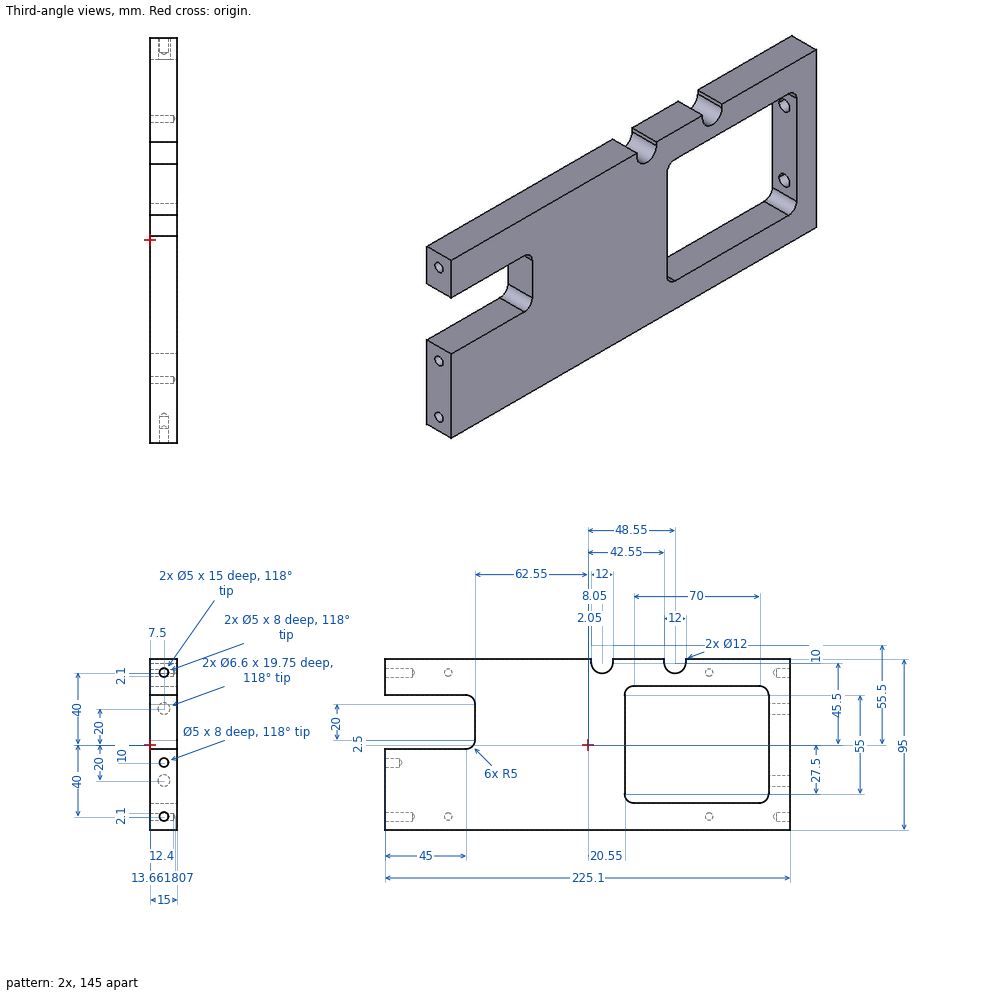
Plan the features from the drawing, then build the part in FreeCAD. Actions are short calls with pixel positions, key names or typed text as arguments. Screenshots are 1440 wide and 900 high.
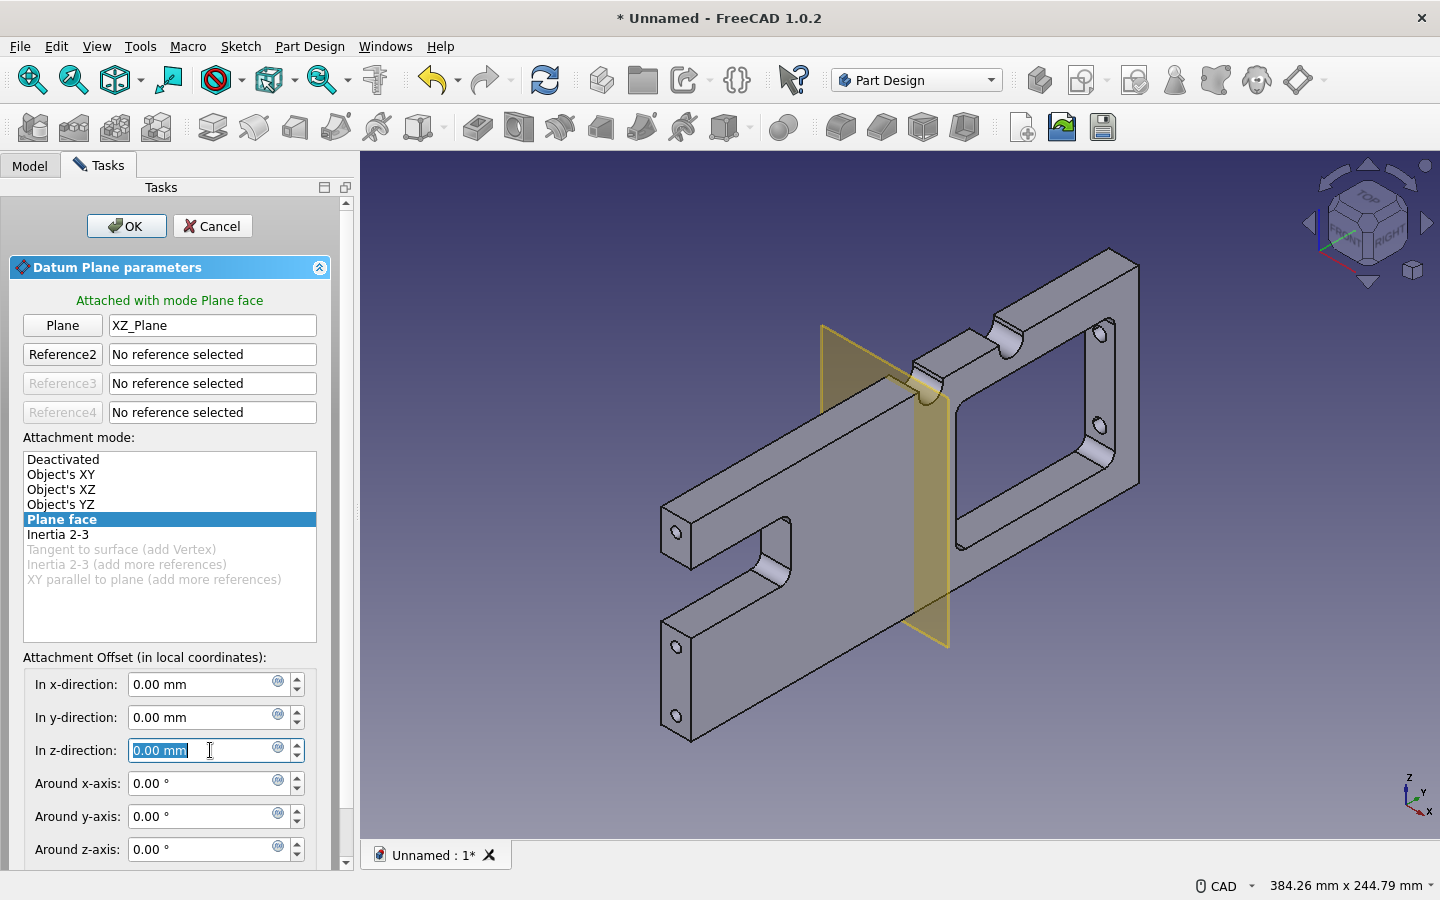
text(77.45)
key(Tab)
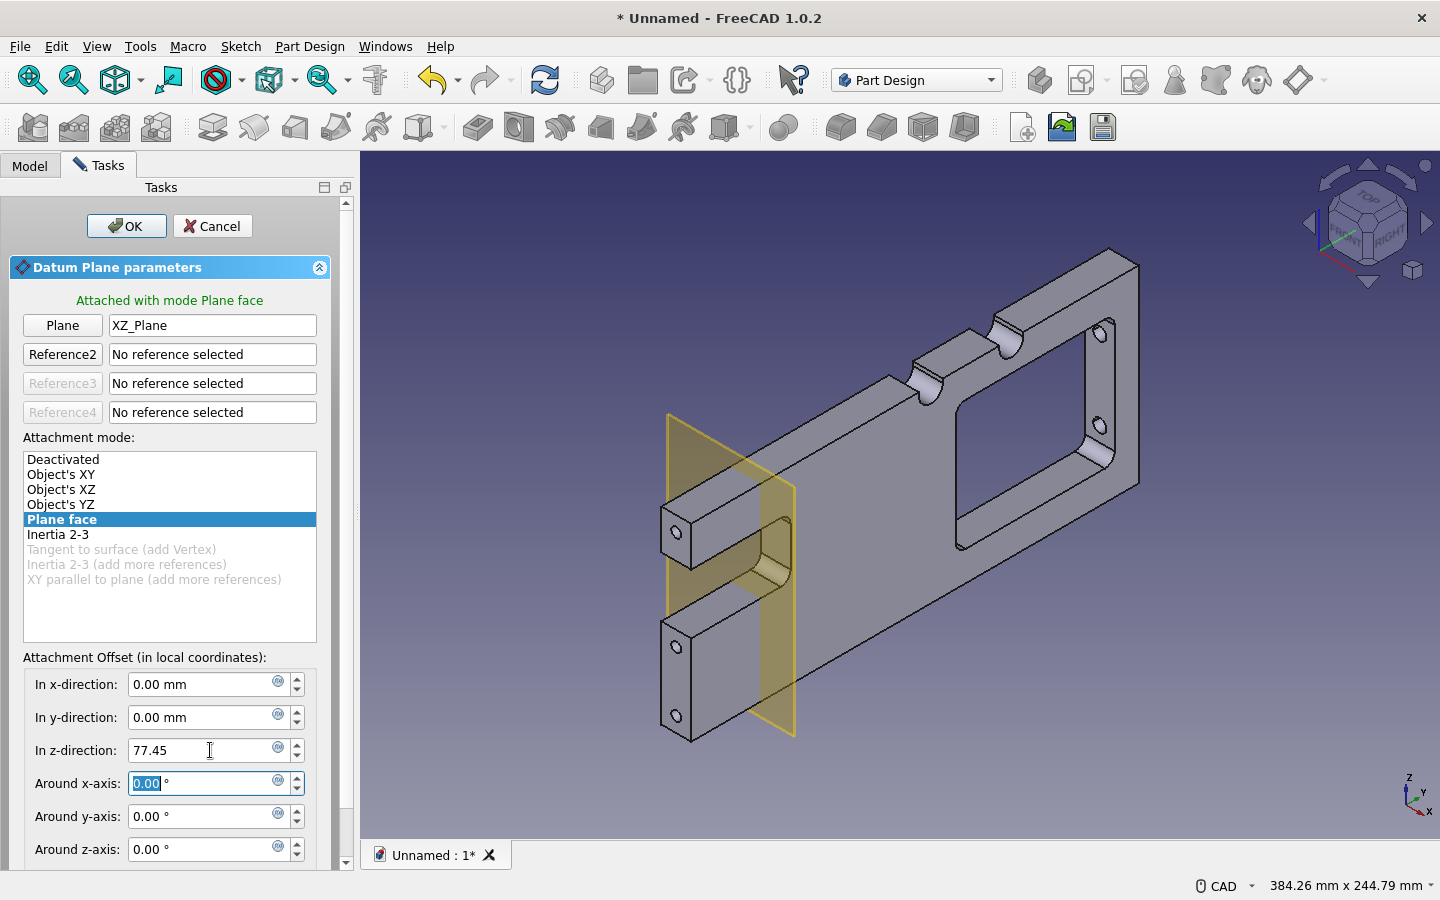
click(127, 226)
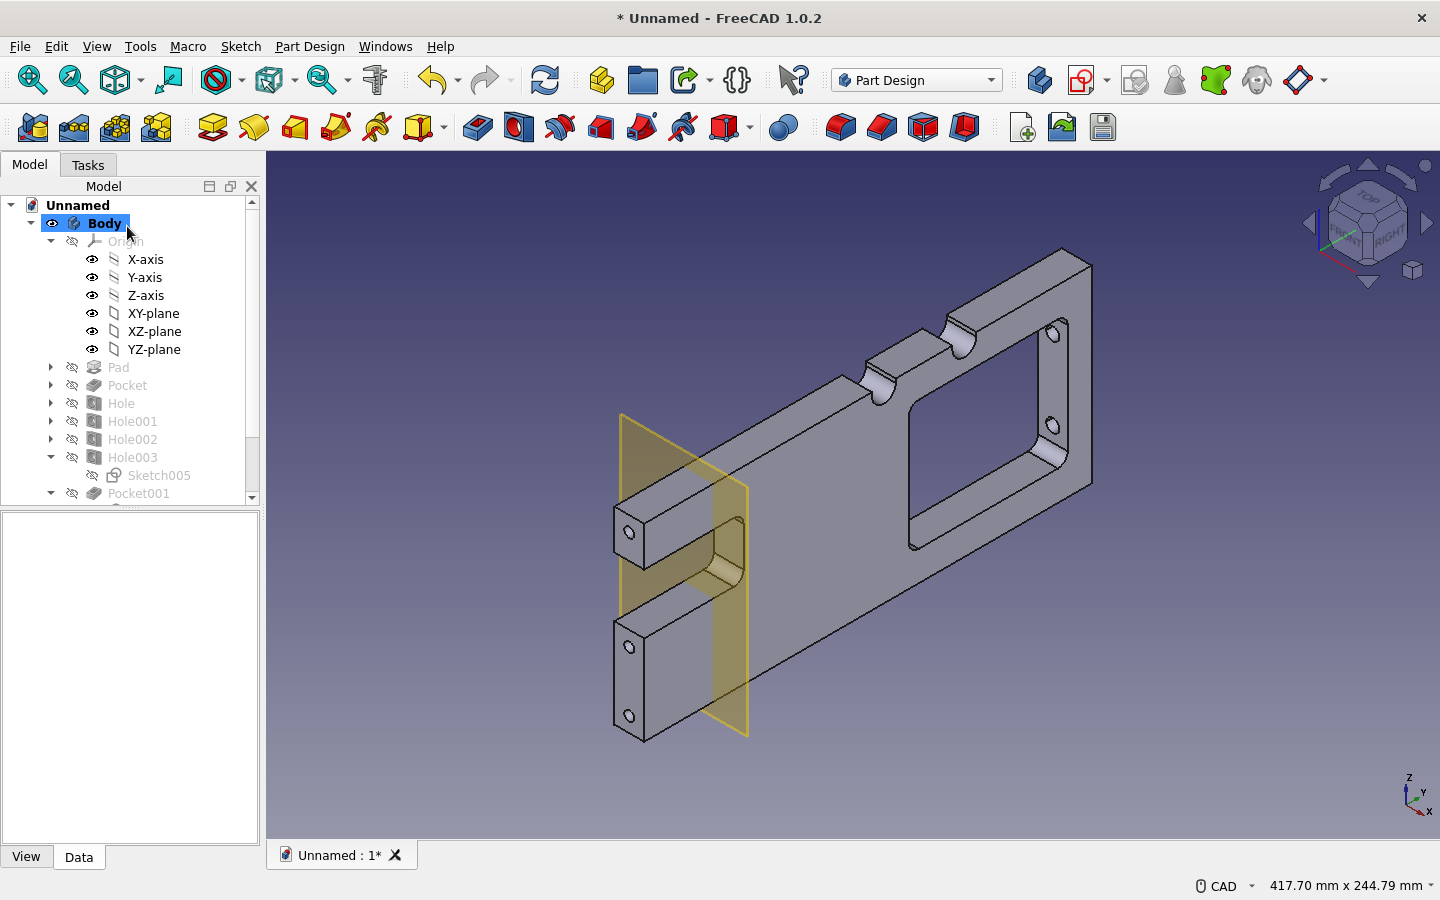
scroll(101, 345, down, 3)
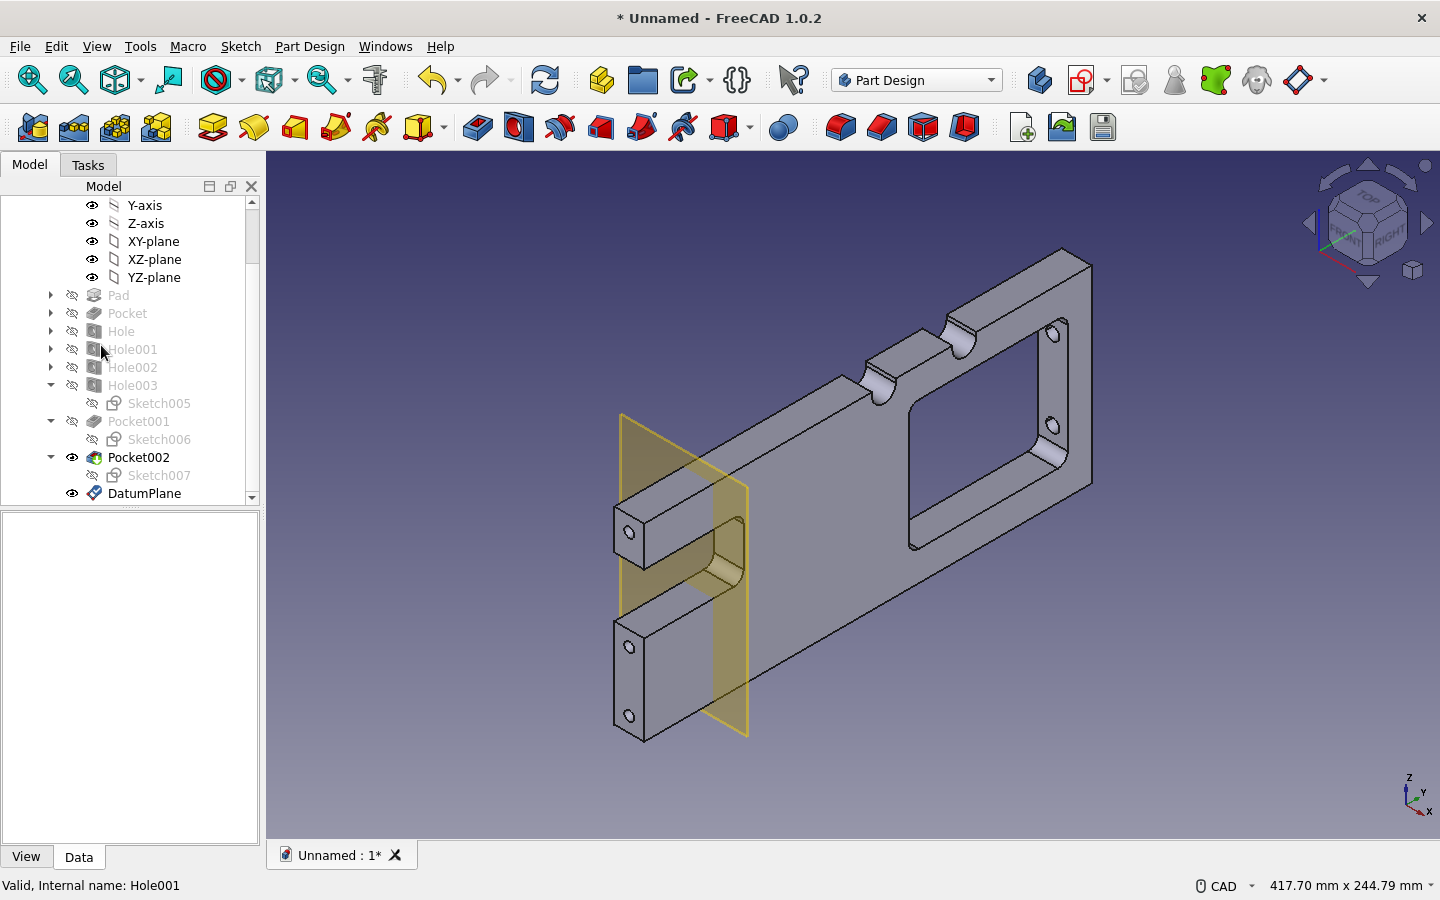
click(117, 493)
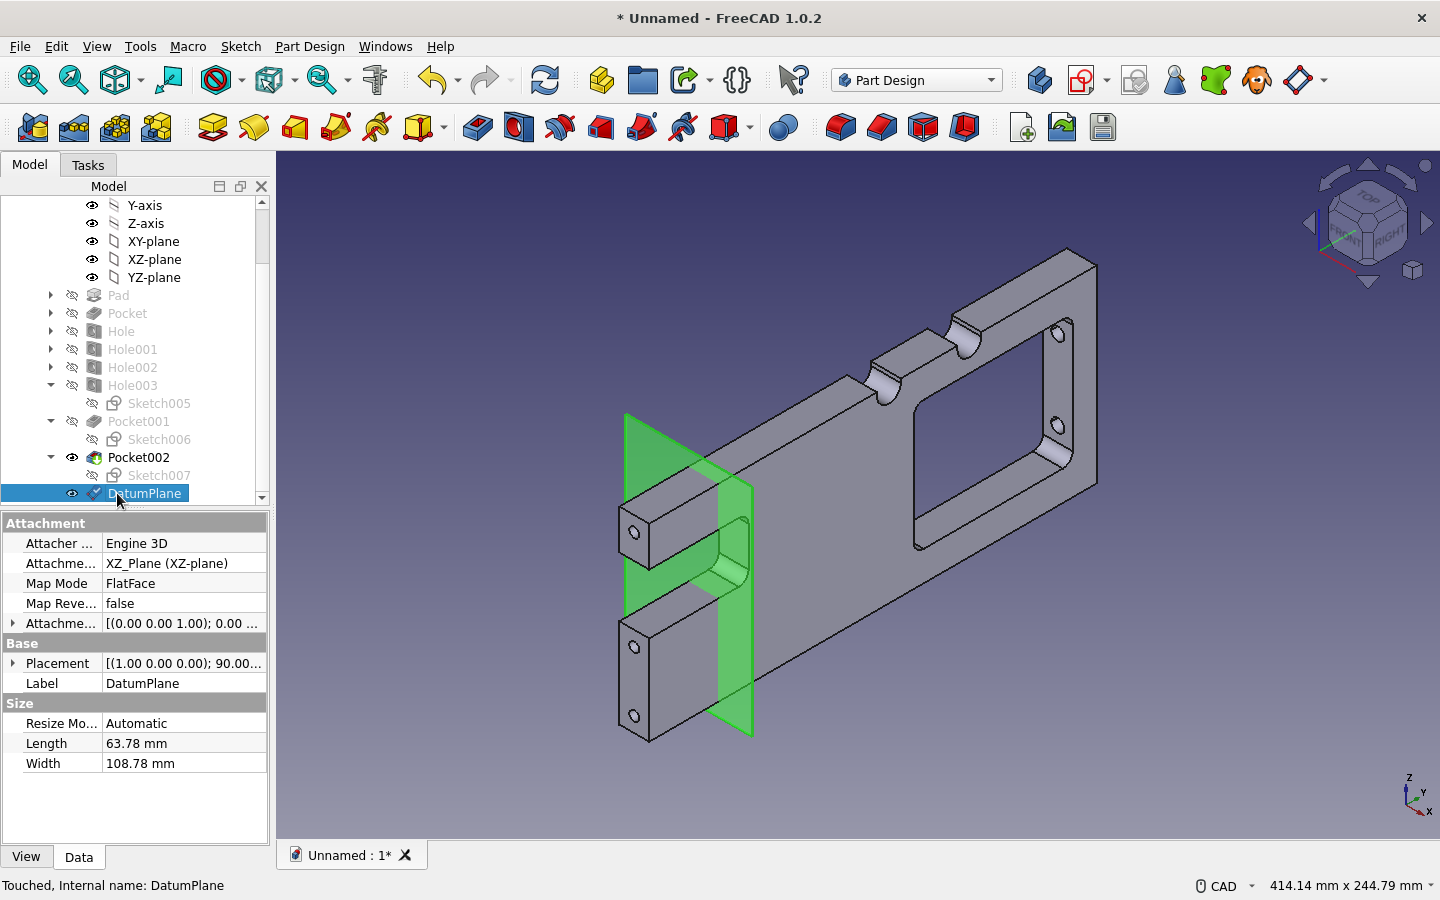
click(1080, 80)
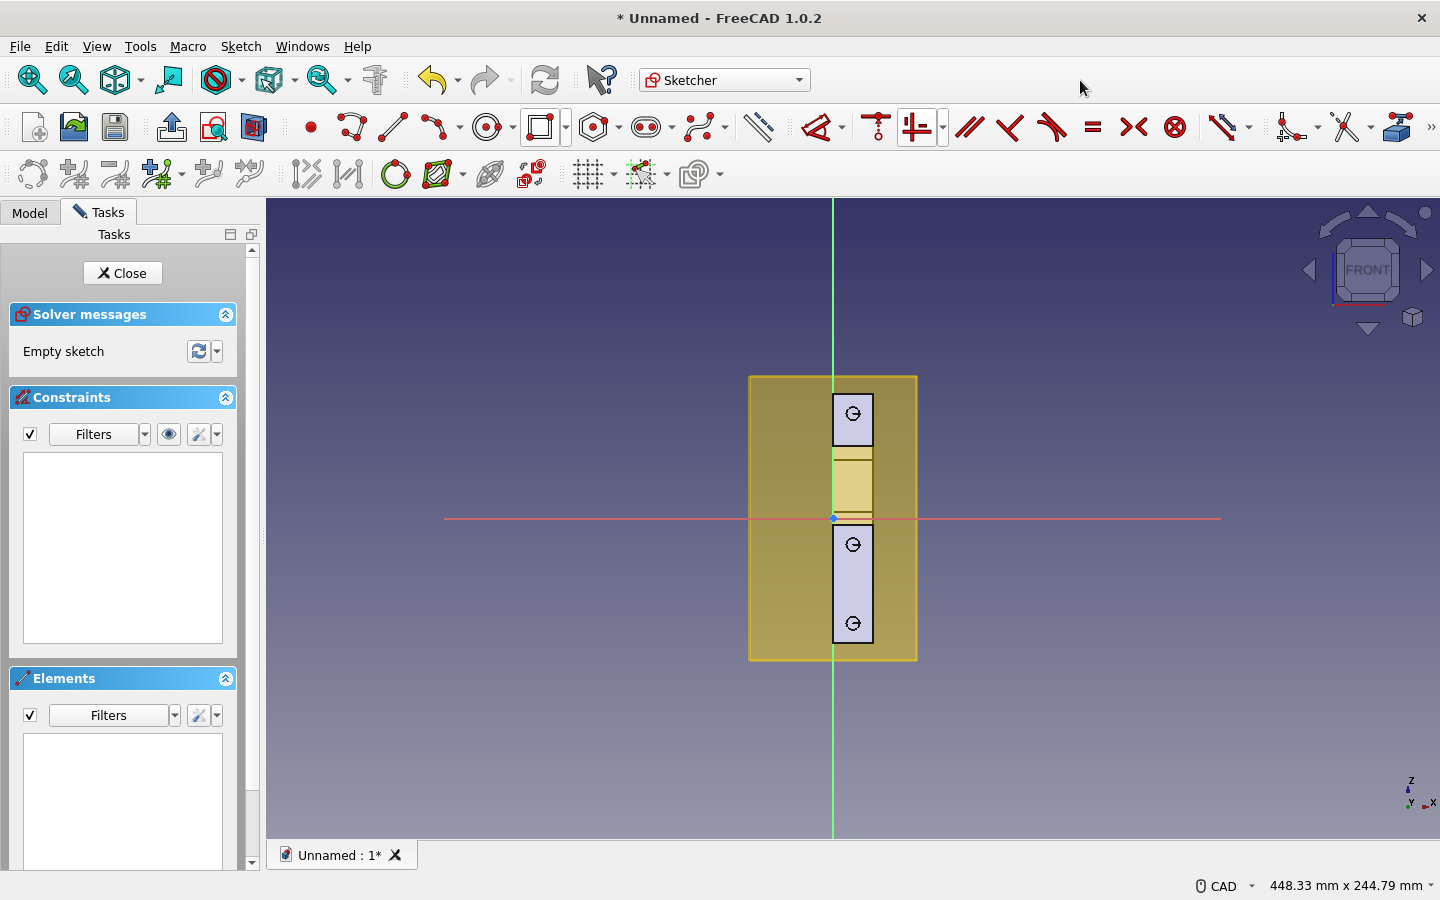
click(254, 128)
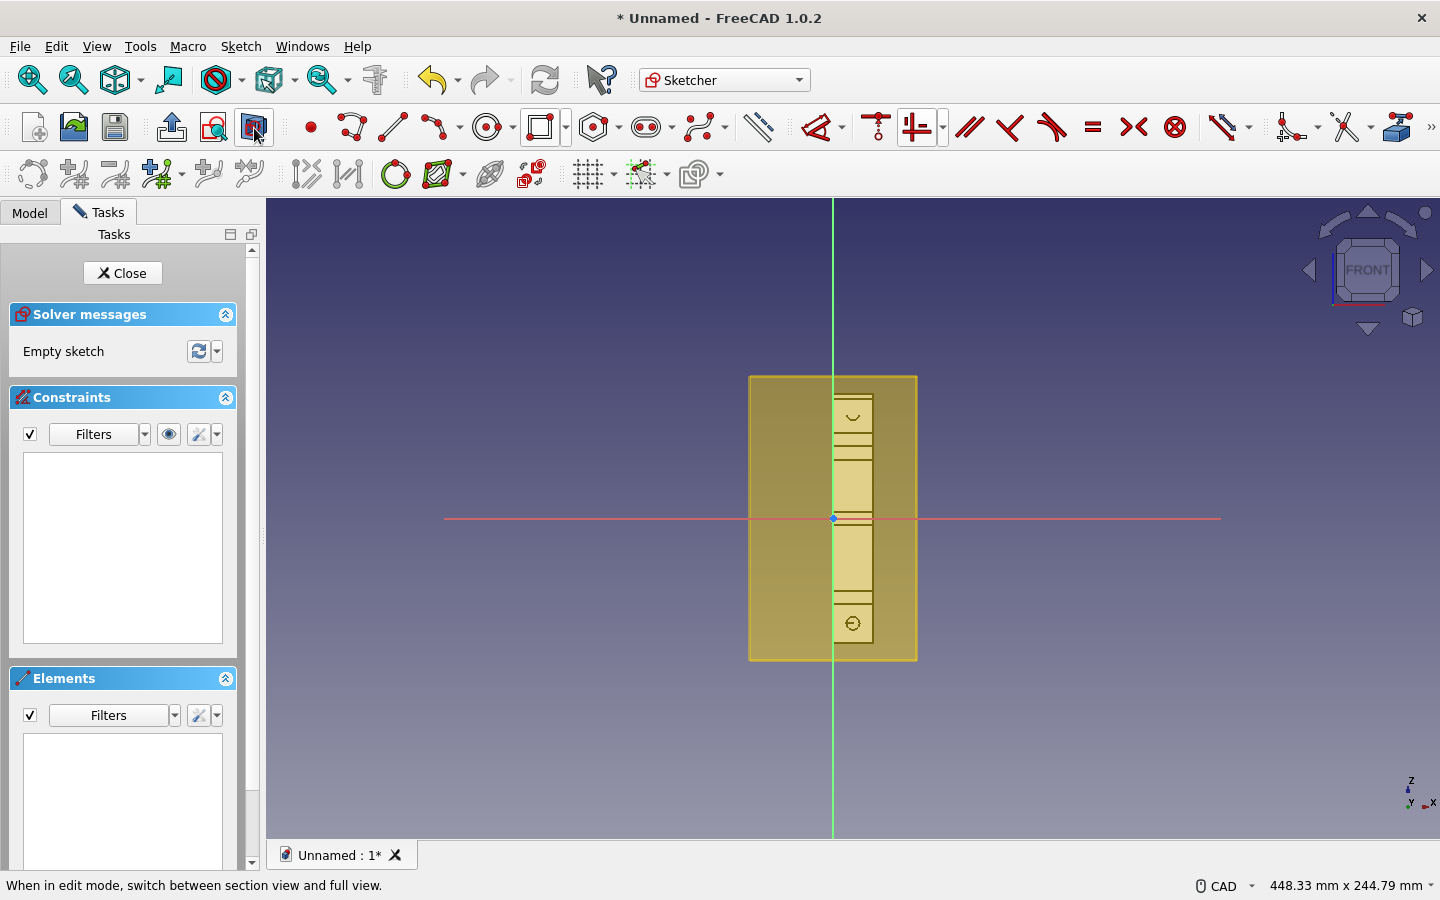
scroll(883, 588, up, 7)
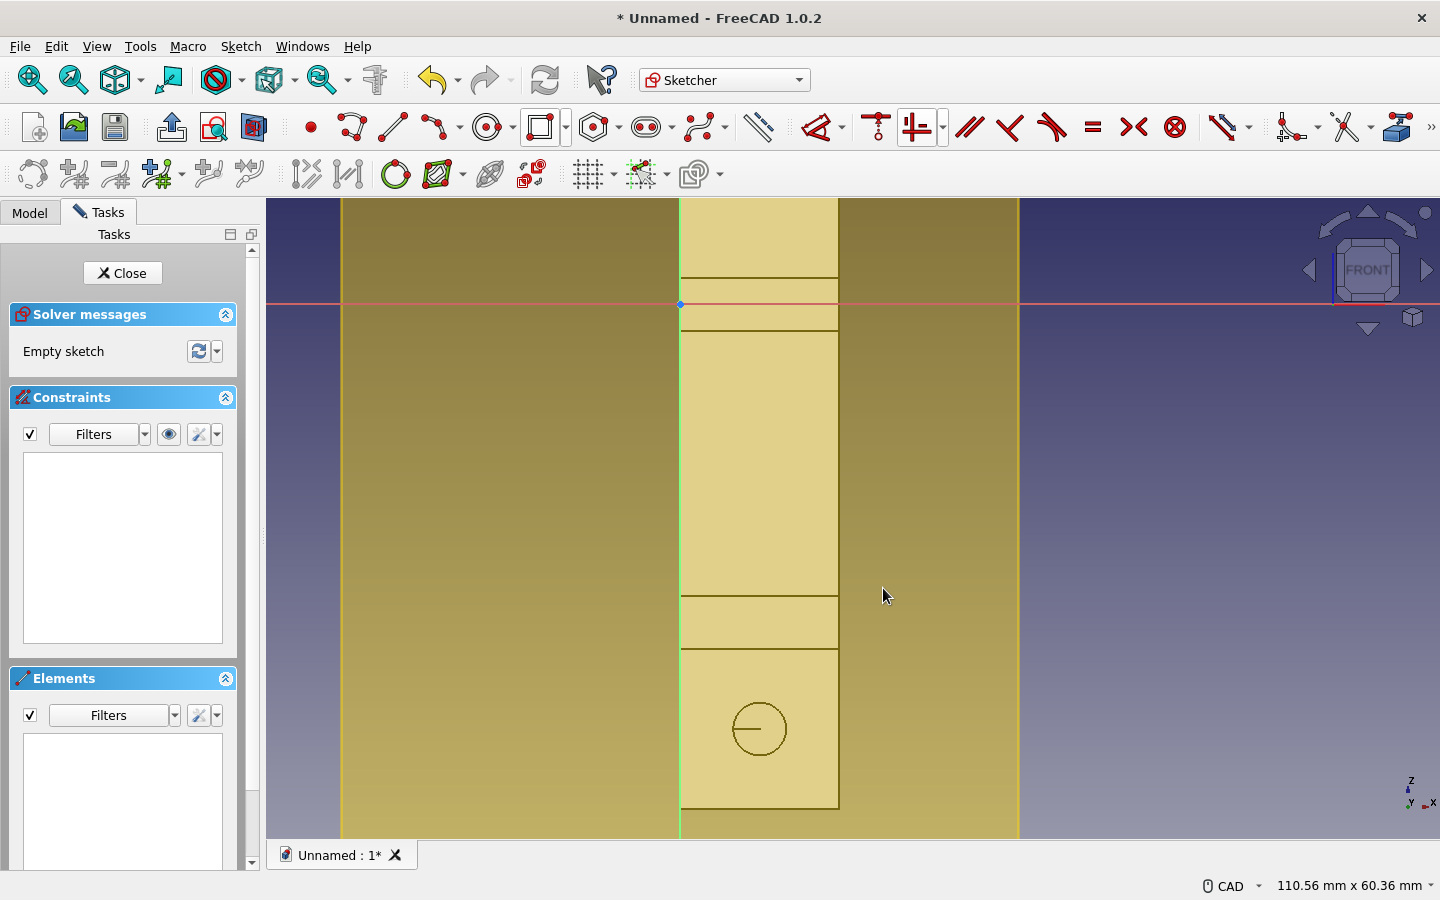
click(352, 128)